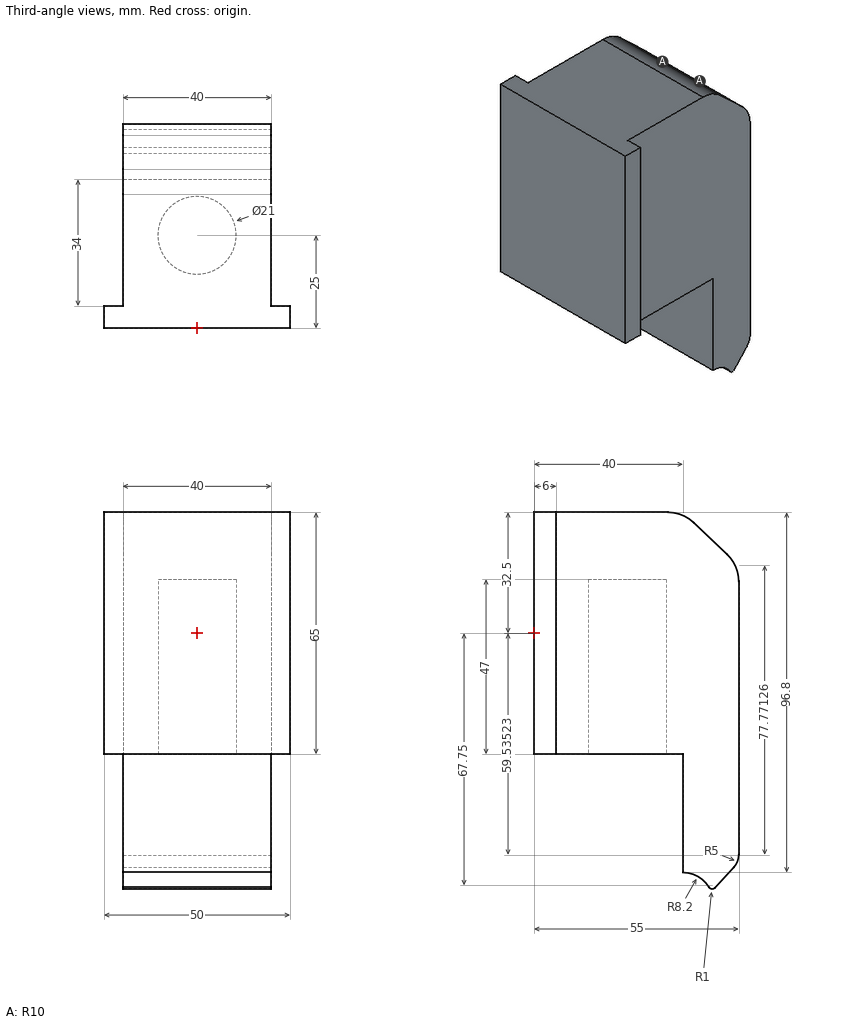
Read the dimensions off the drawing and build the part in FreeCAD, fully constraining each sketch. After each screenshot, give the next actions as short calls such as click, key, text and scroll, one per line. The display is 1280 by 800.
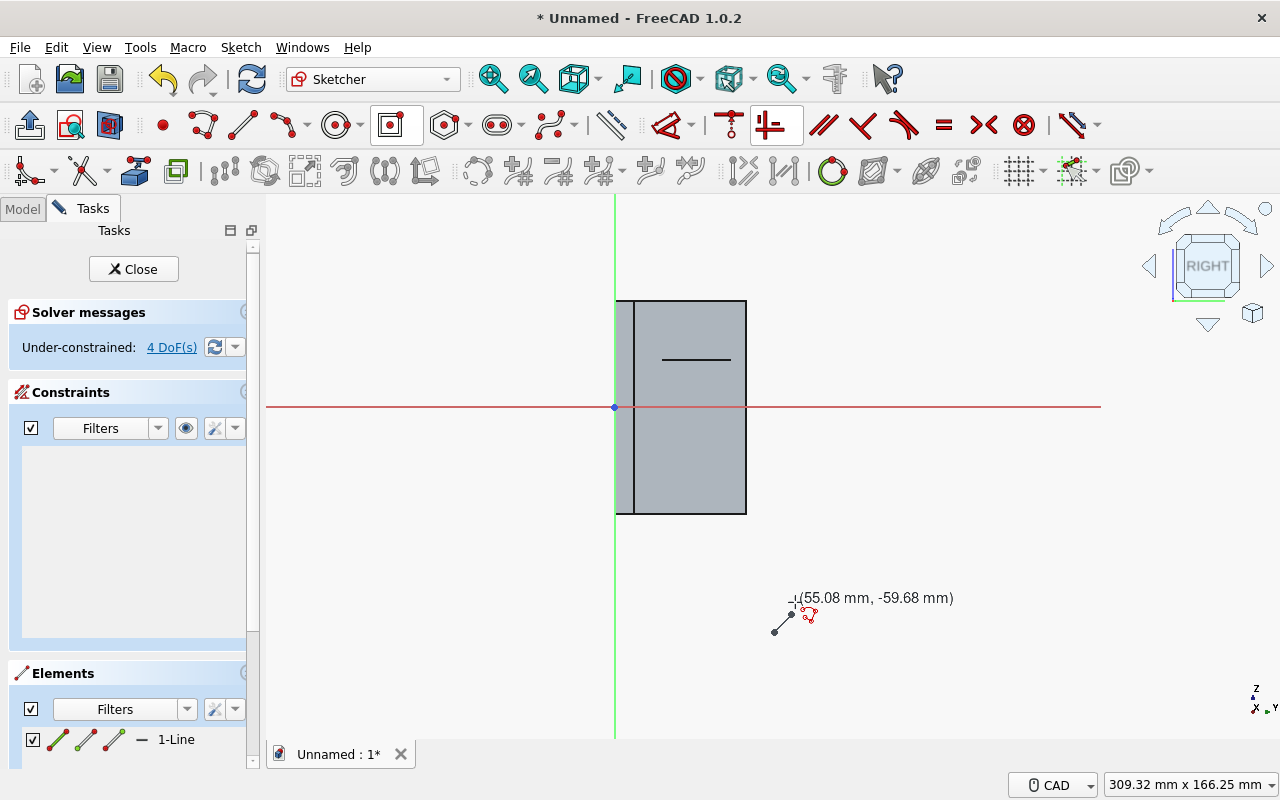
click(795, 348)
click(746, 301)
click(746, 618)
right_click(746, 618)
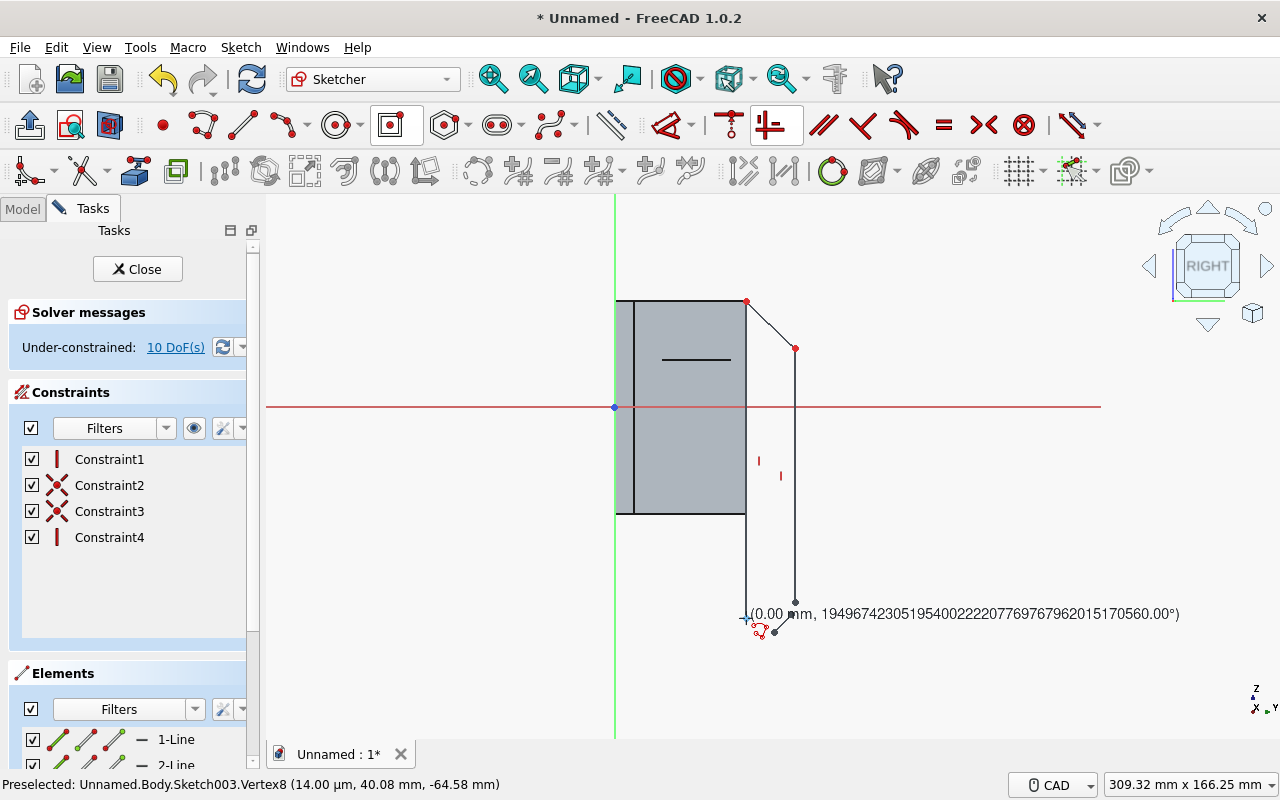
click(284, 126)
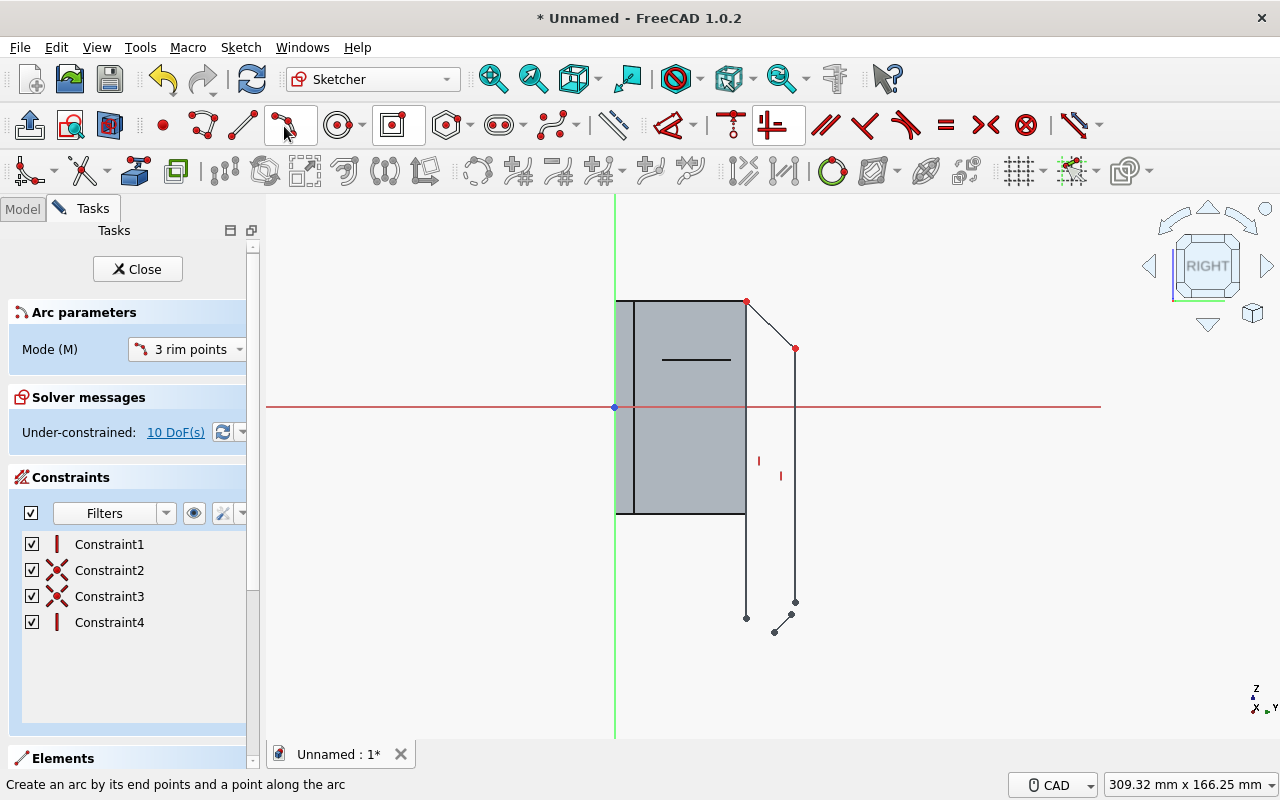
scroll(791, 614, up, 2)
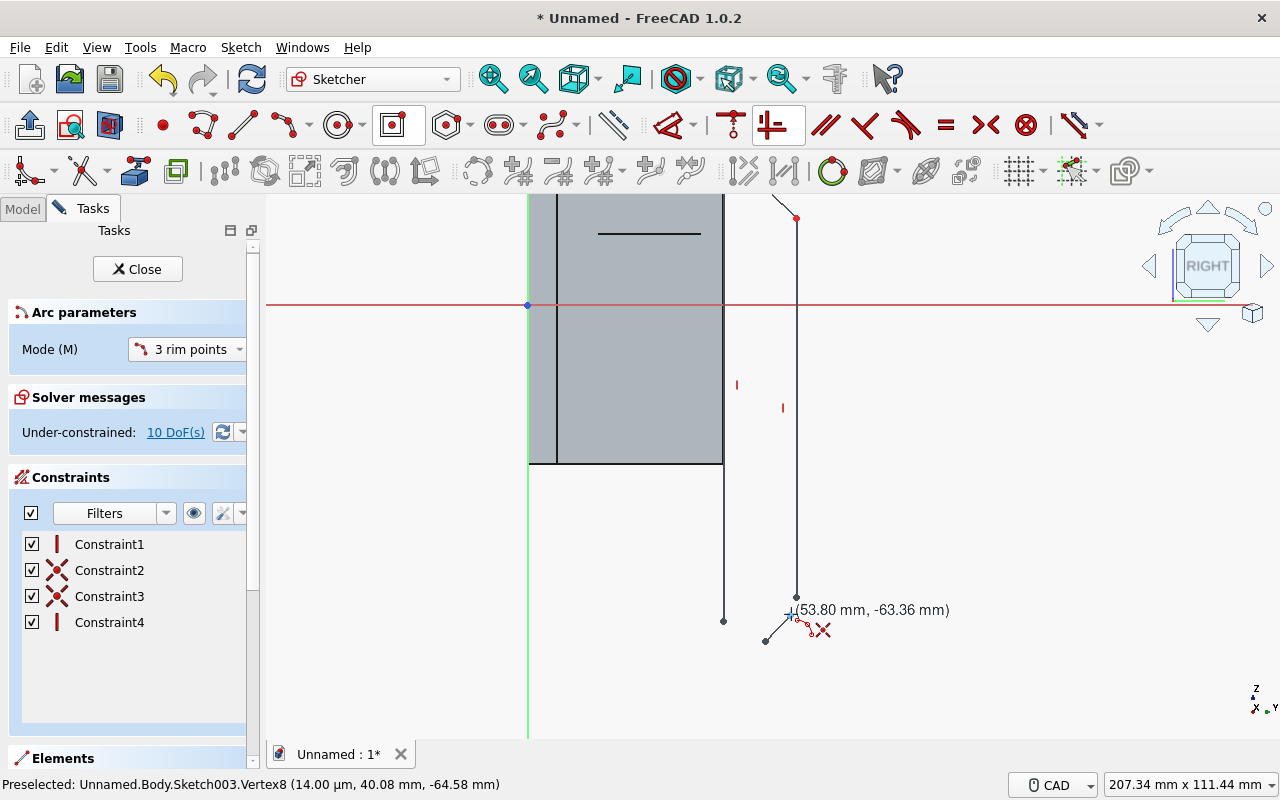
click(791, 615)
click(797, 597)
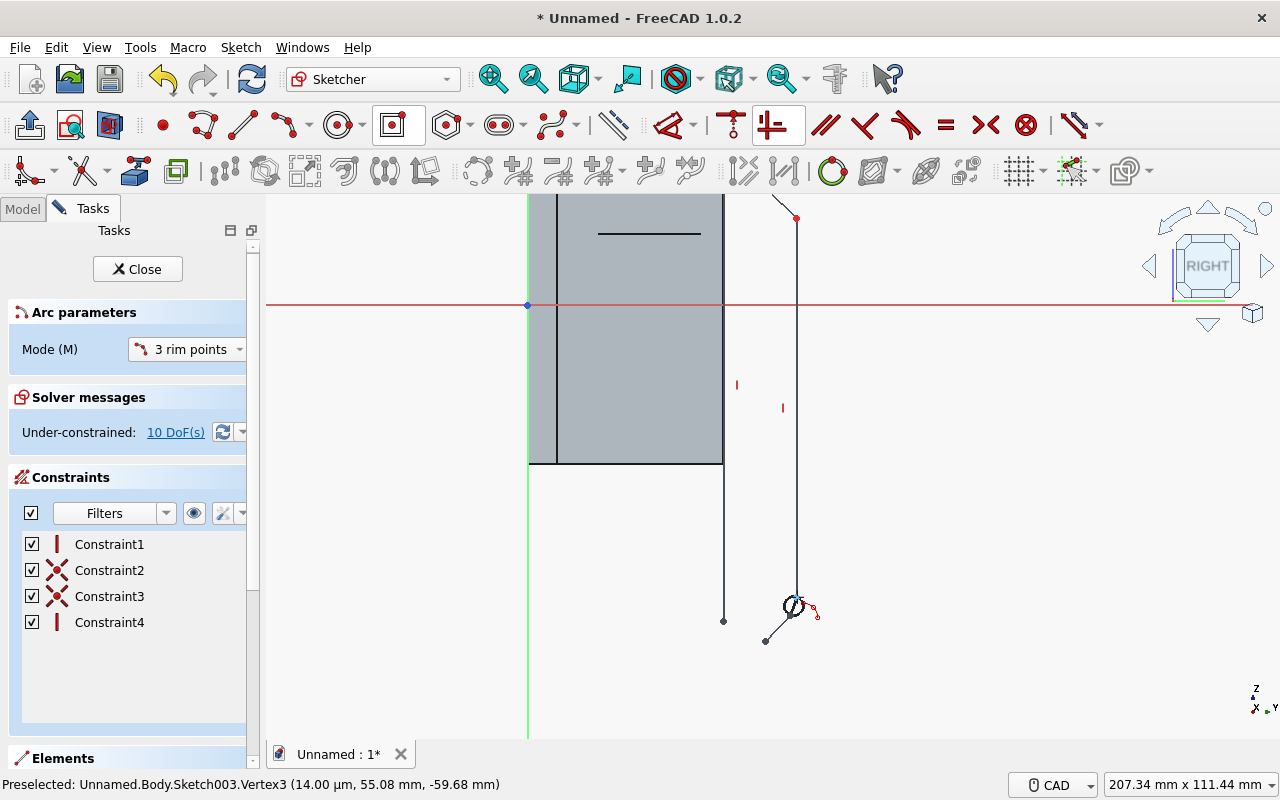
scroll(795, 605, up, 12)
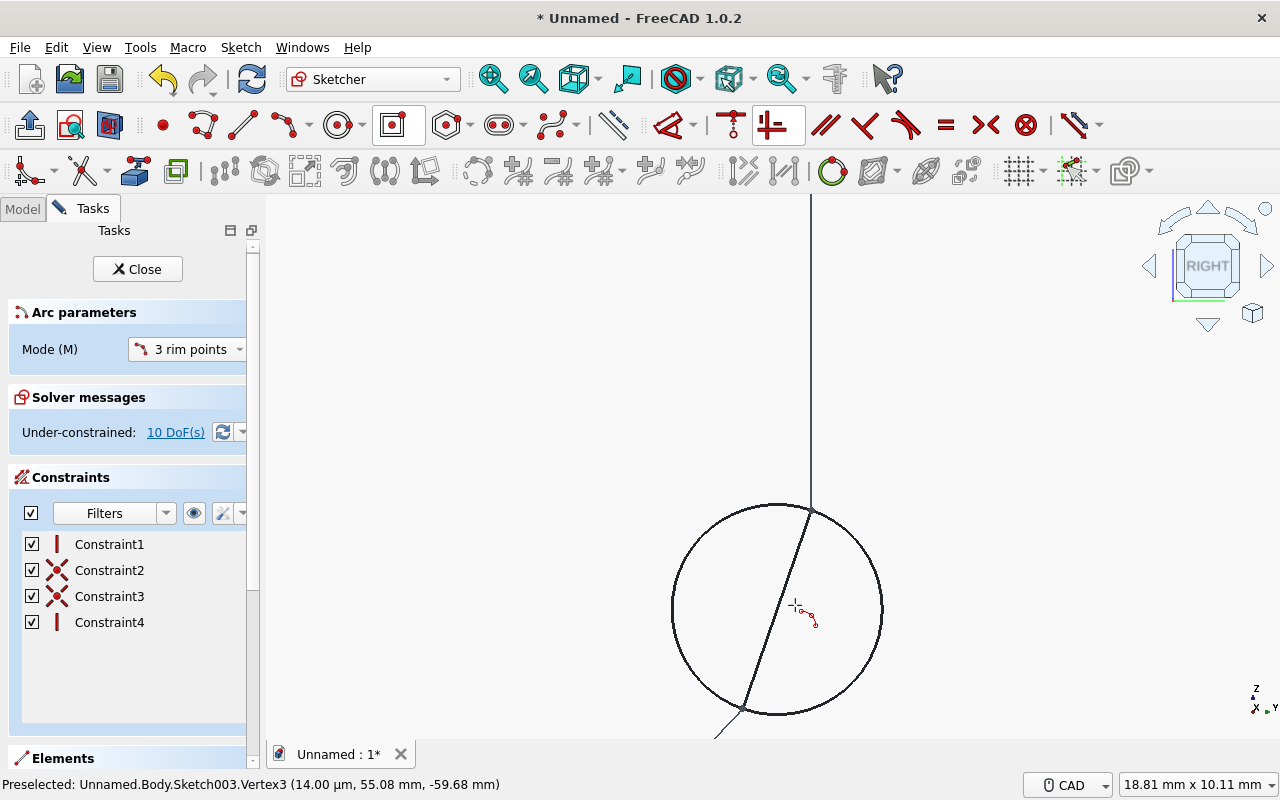
click(789, 600)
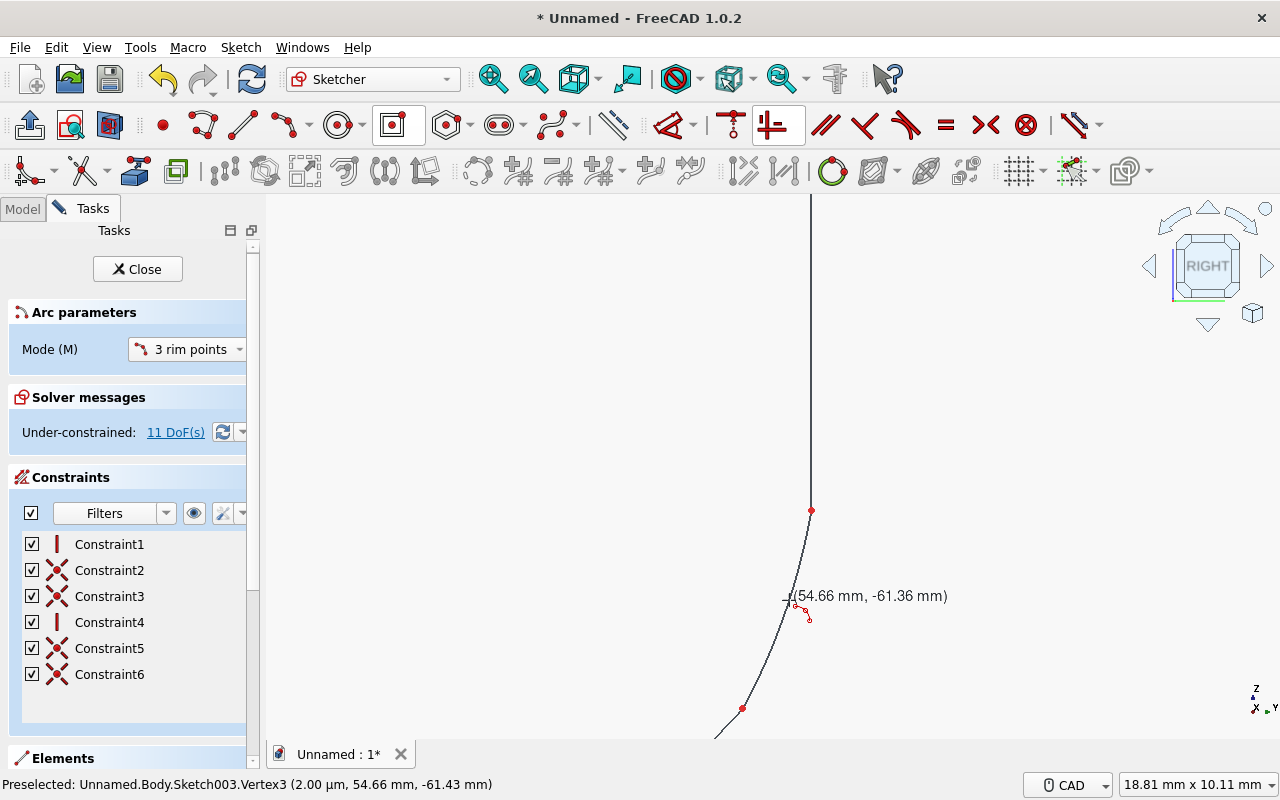
scroll(794, 609, down, 14)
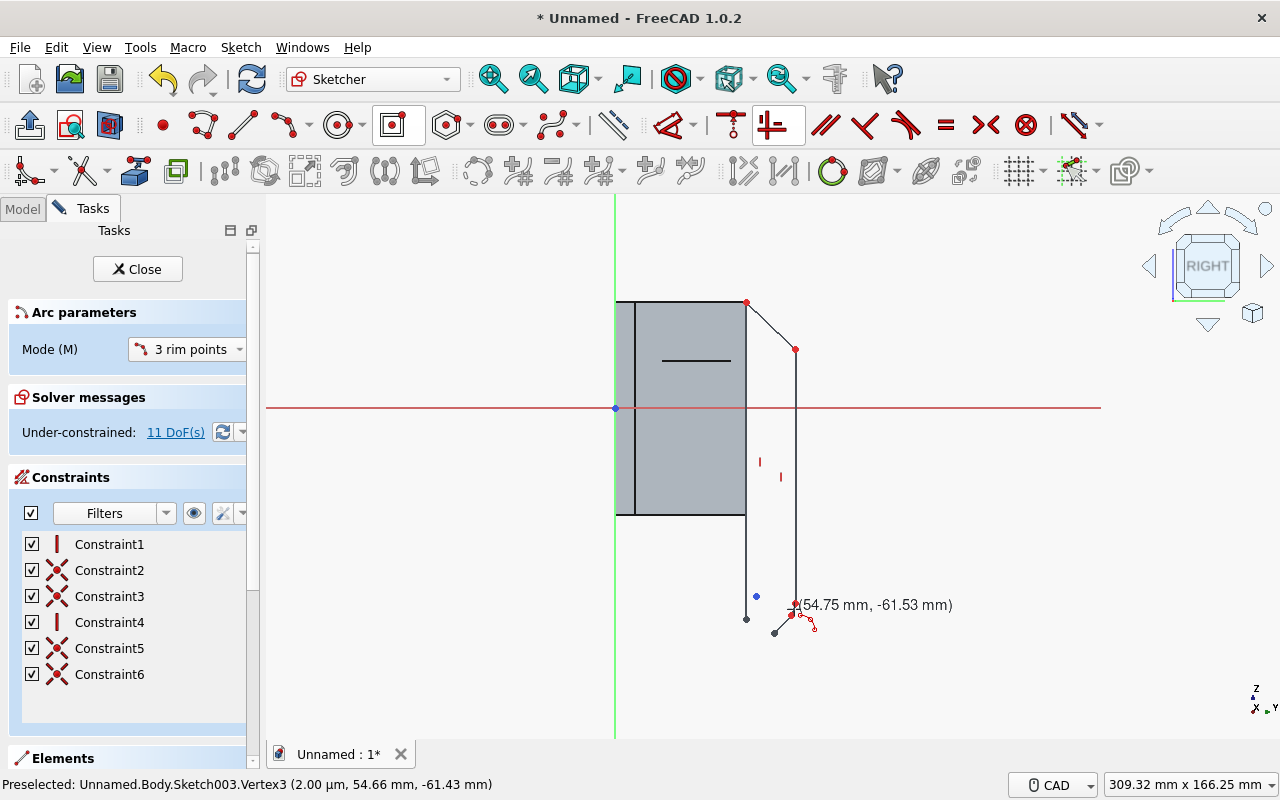
click(746, 620)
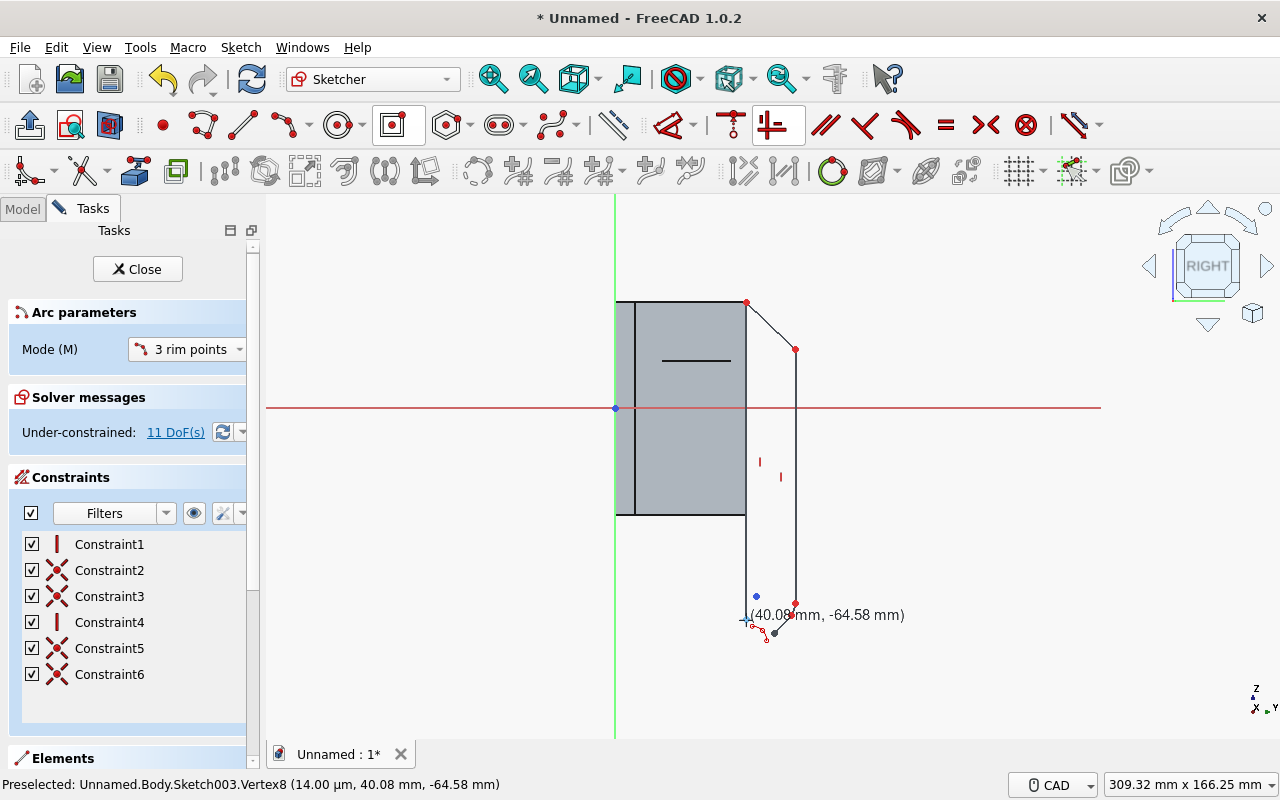
scroll(769, 632, up, 6)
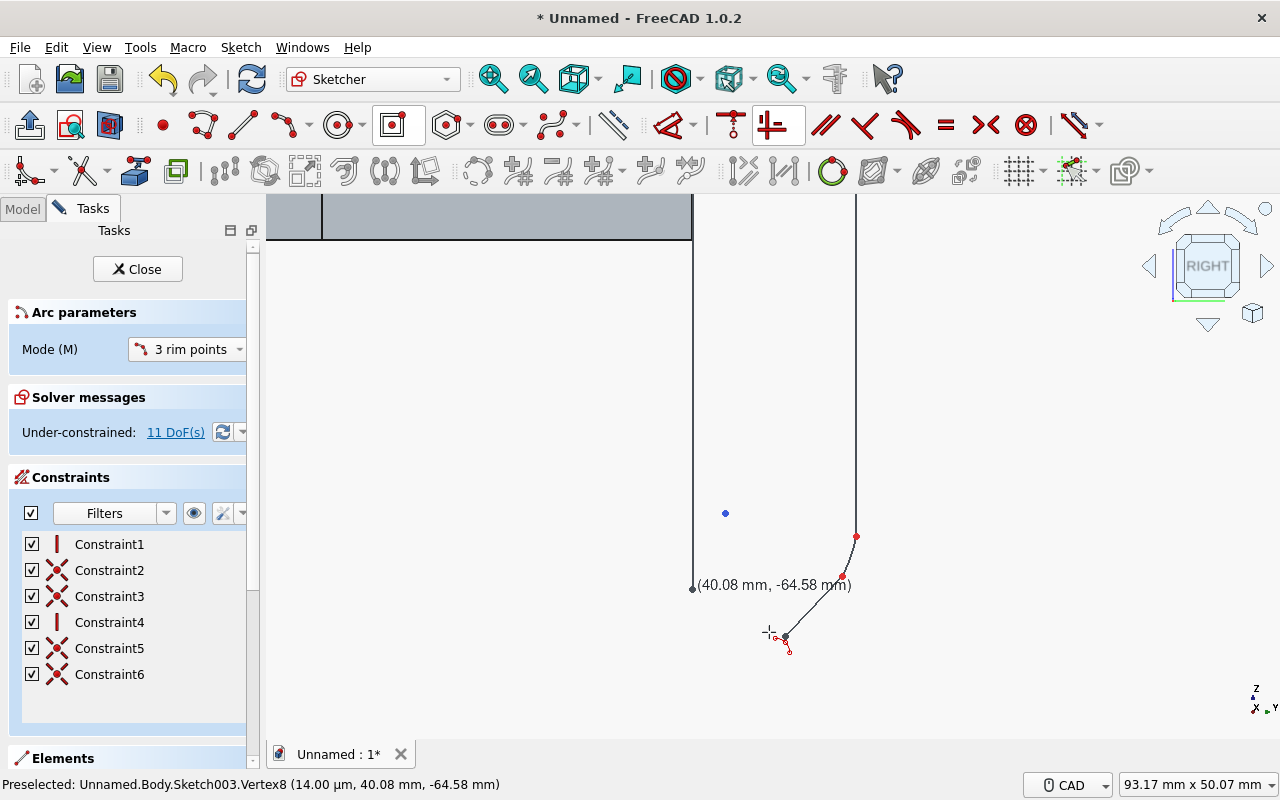
click(768, 630)